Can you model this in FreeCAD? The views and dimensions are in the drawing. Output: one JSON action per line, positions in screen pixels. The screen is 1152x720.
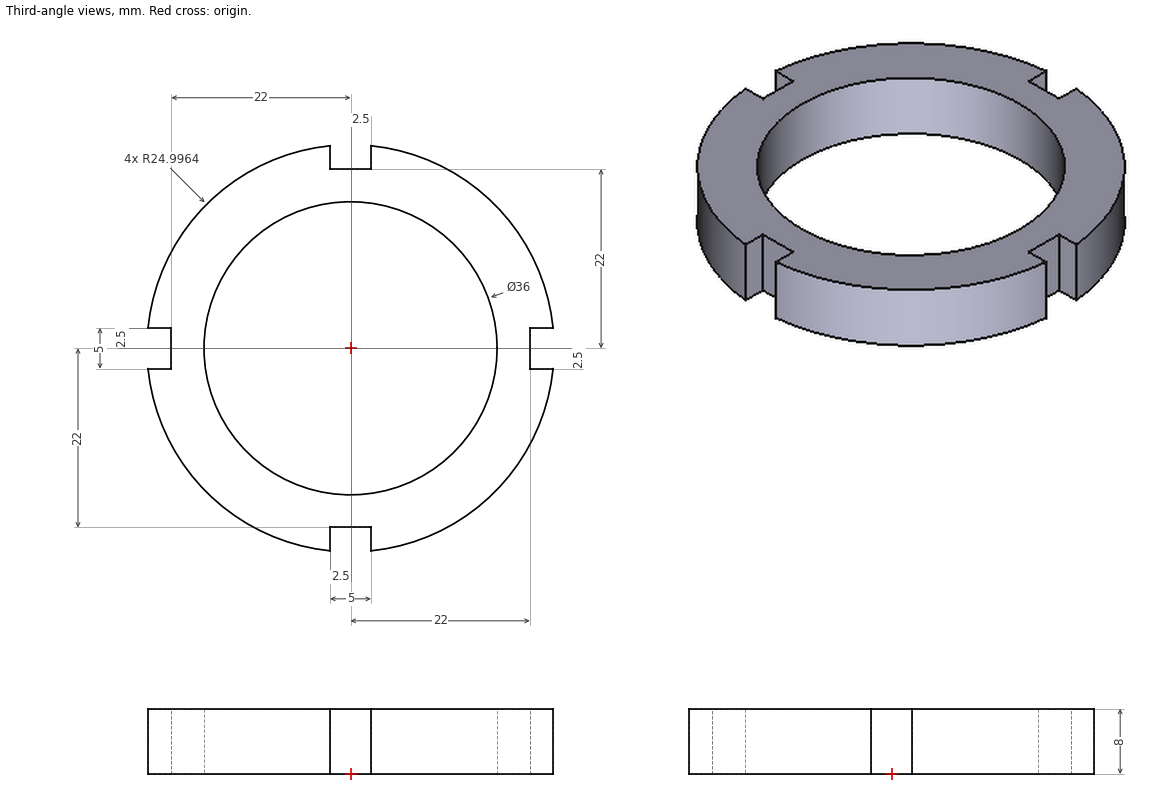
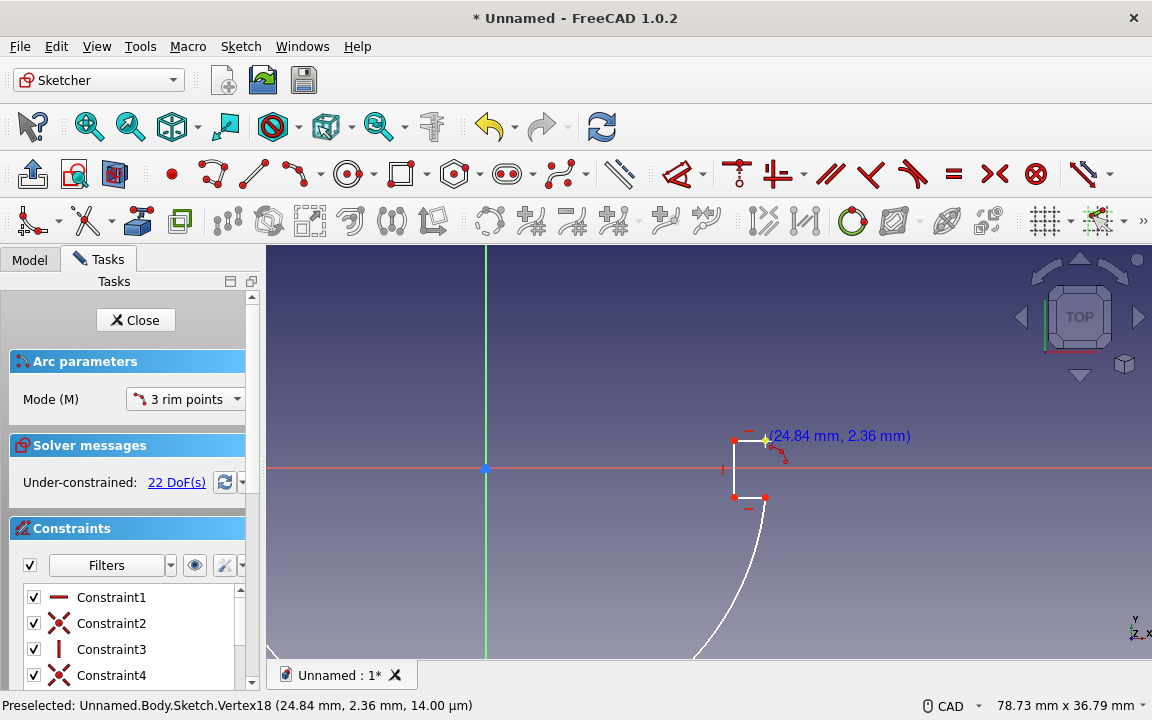
{"action": "scroll", "coordinate": [767, 439], "scroll_direction": "down", "scroll_amount": 4}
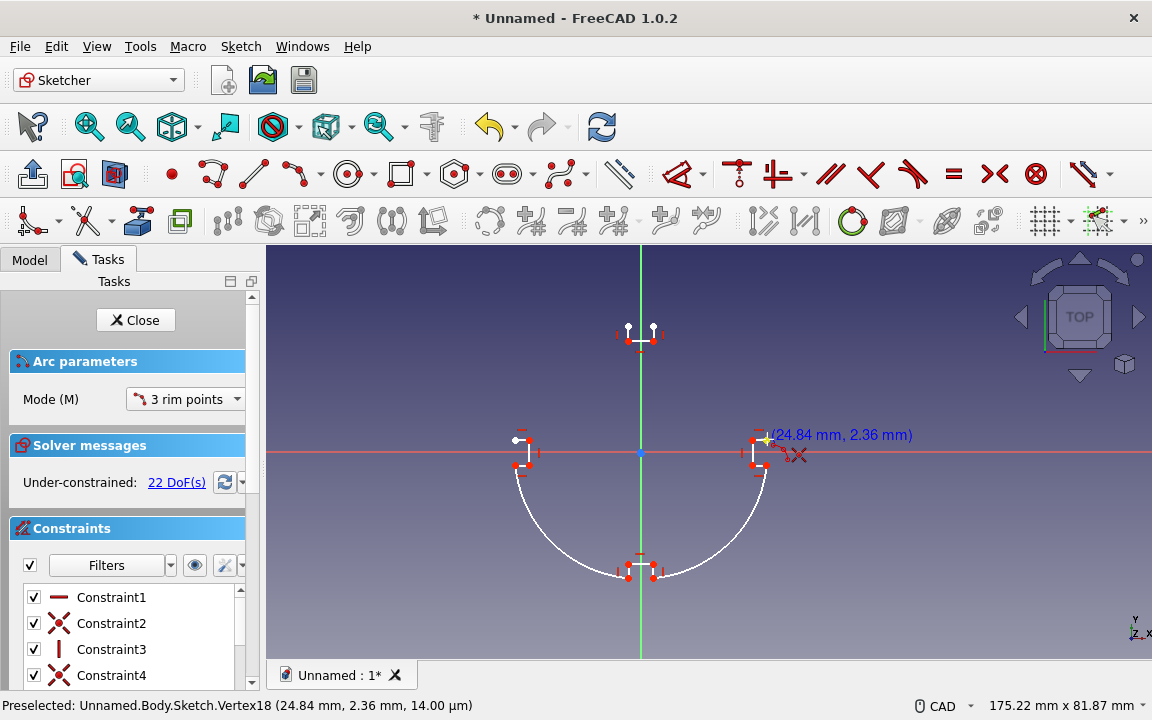
{"action": "scroll", "coordinate": [654, 326], "scroll_direction": "up", "scroll_amount": 4}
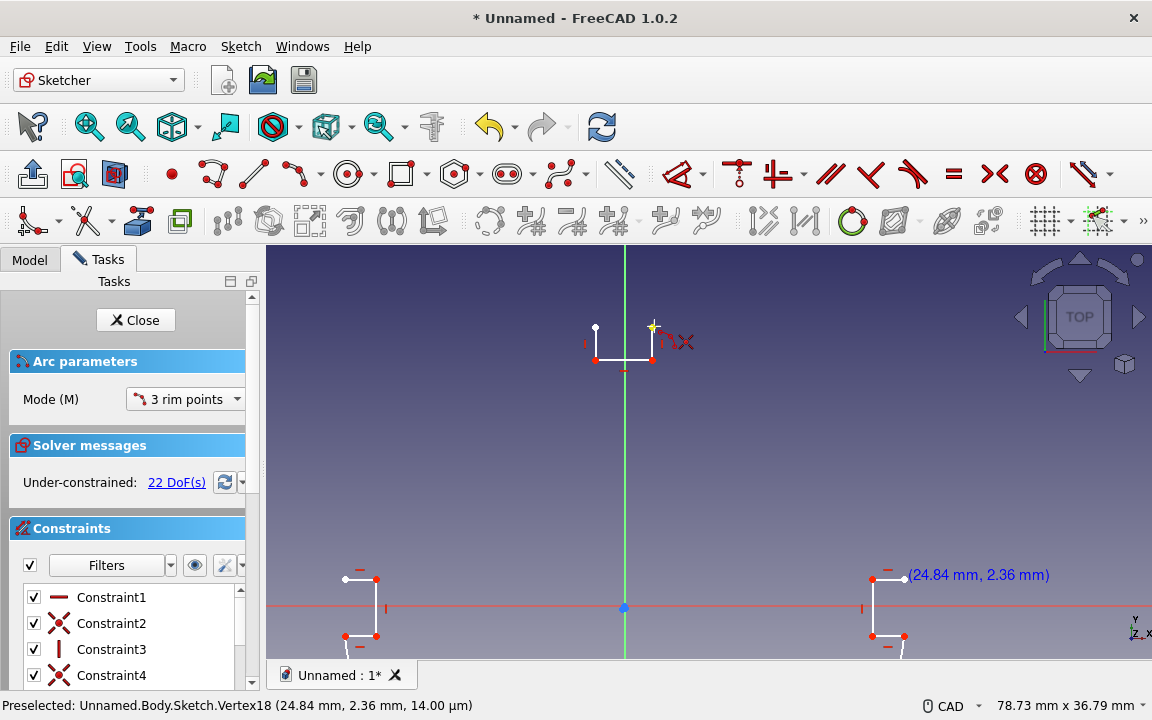
{"action": "left_click", "coordinate": [652, 327]}
{"action": "left_click", "coordinate": [823, 407]}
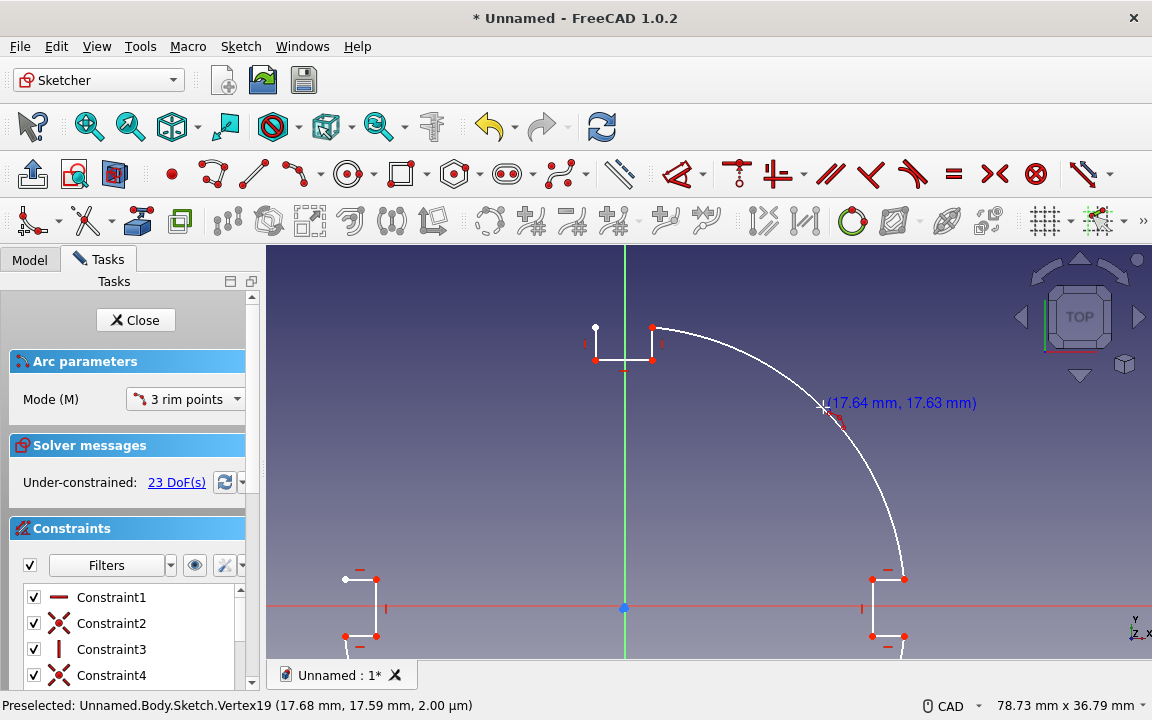
{"action": "left_click", "coordinate": [596, 327]}
{"action": "left_click", "coordinate": [345, 580]}
{"action": "left_click", "coordinate": [426, 407]}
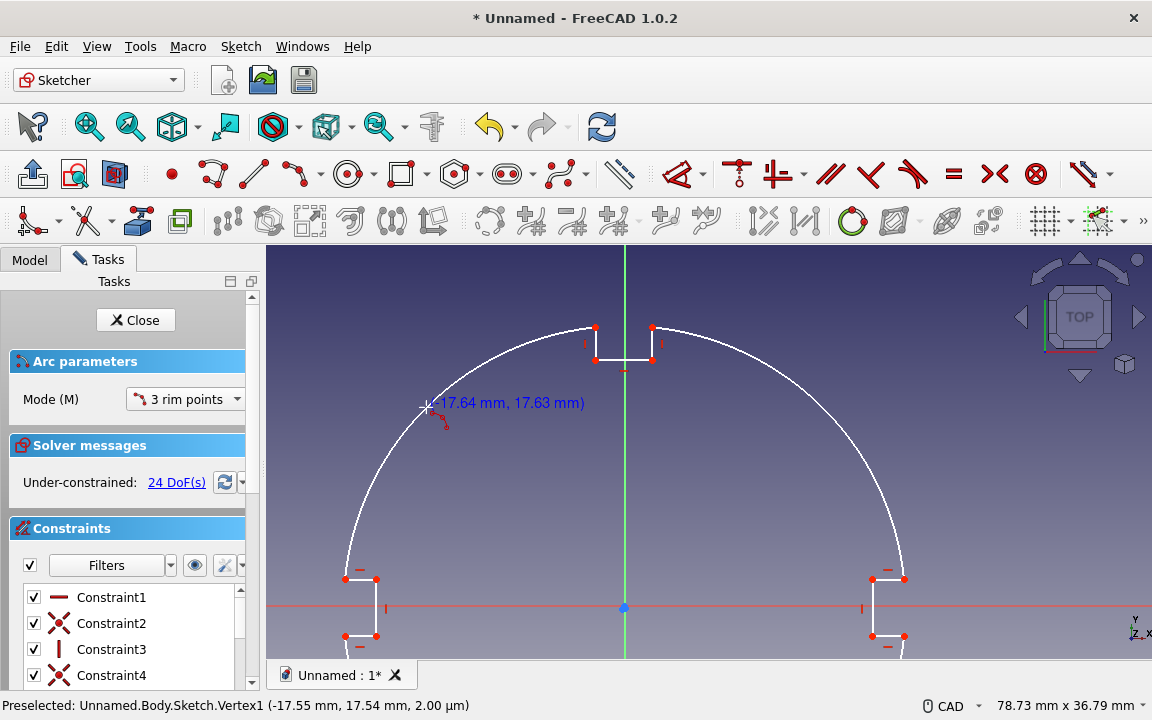
{"action": "key", "text": "g c"}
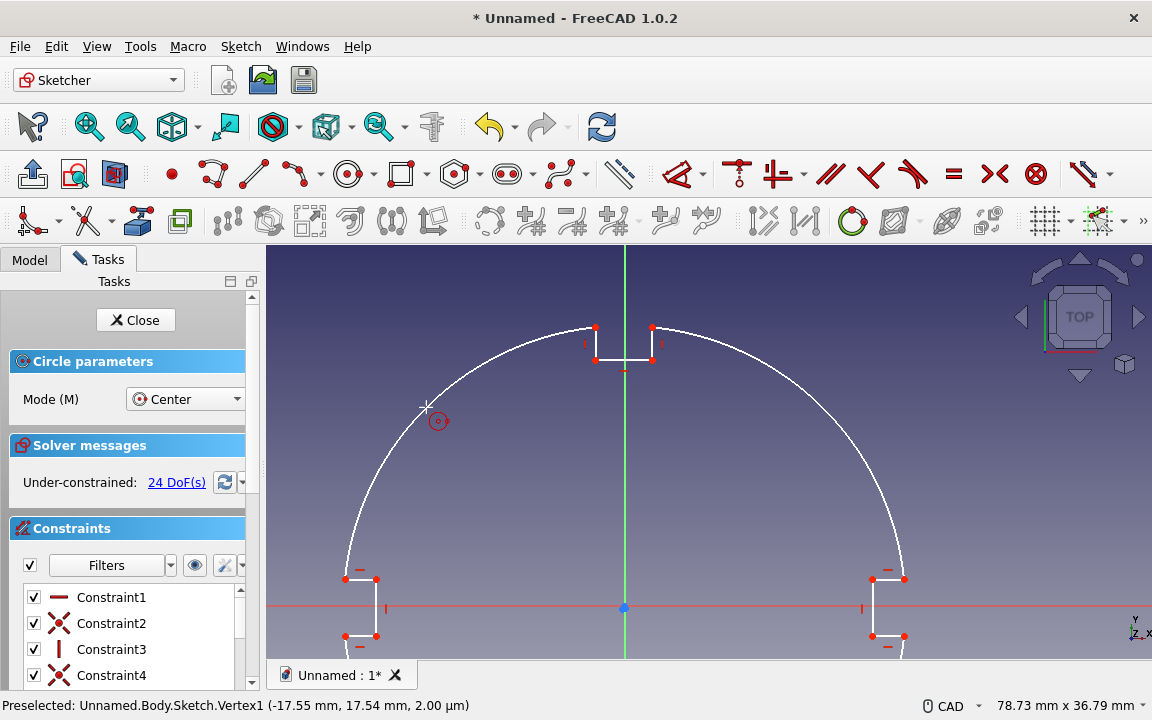
{"action": "left_click", "coordinate": [625, 606]}
{"action": "mouse_move", "coordinate": [768, 463]}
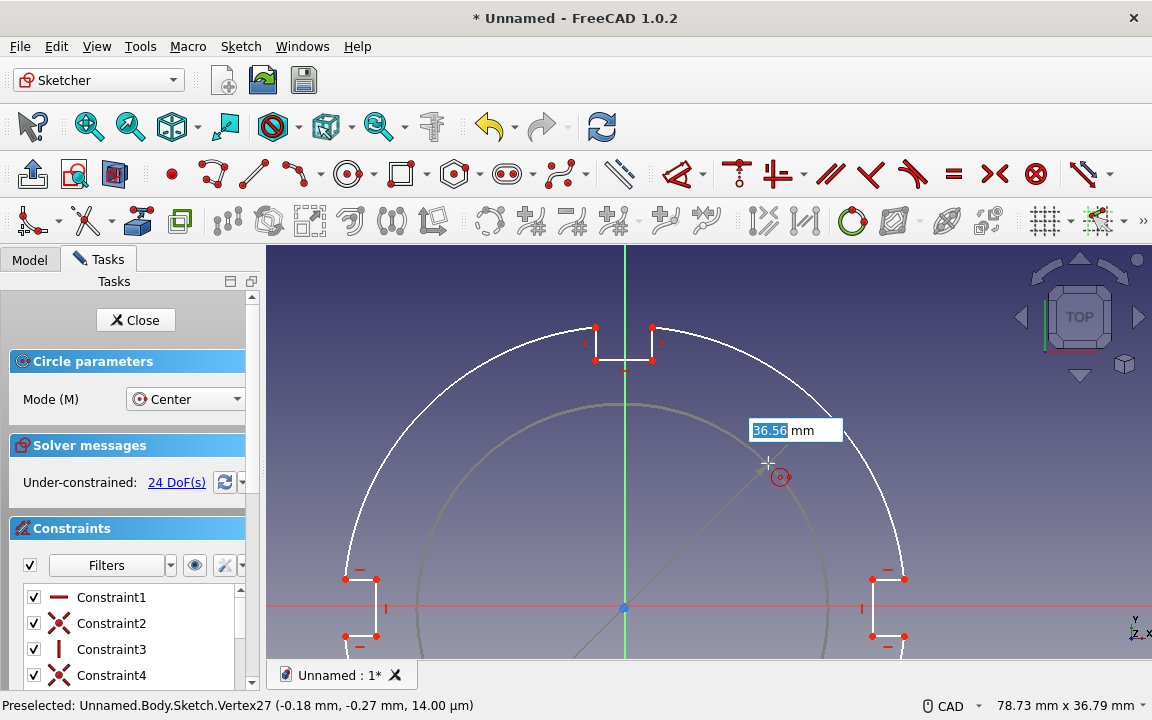
{"action": "type", "text": "36"}
{"action": "key", "text": "Return"}
{"action": "key", "text": "Escape"}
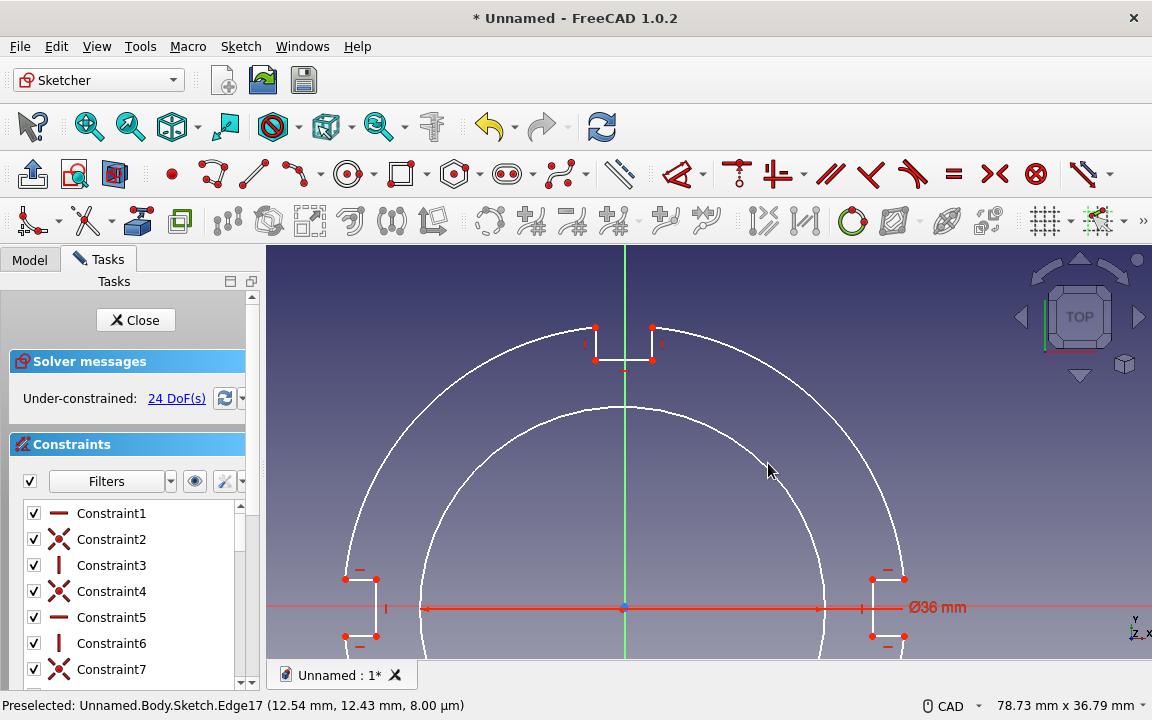
{"action": "left_click", "coordinate": [765, 466]}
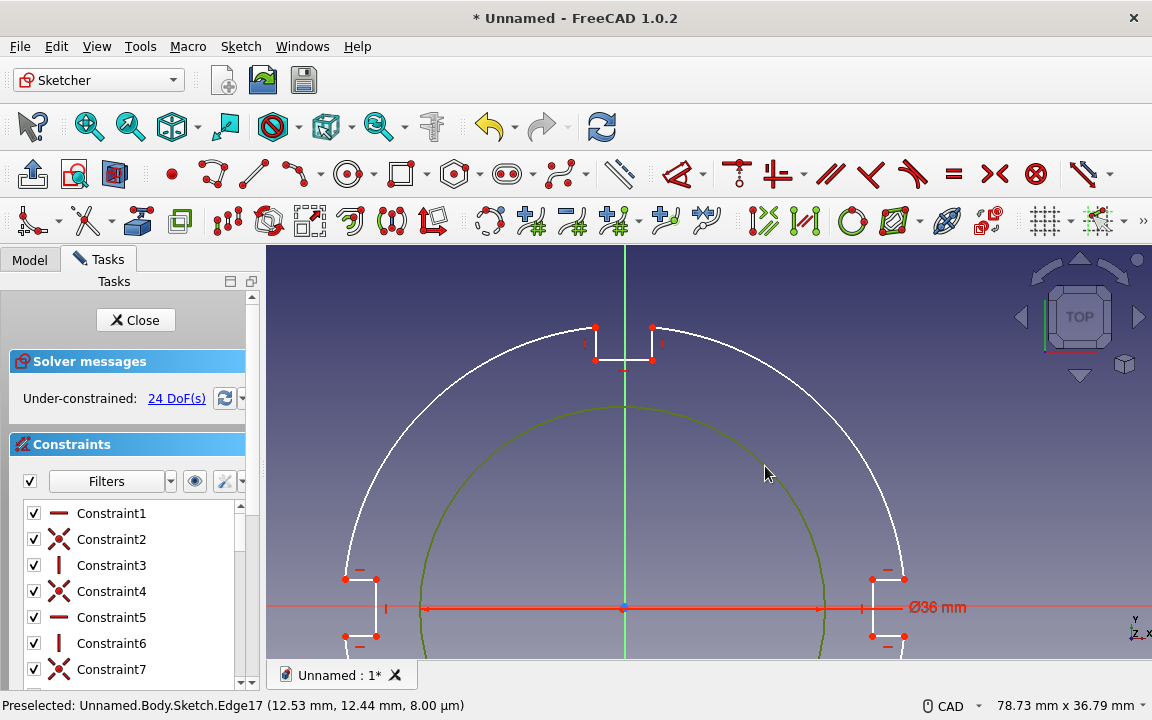
{"action": "scroll", "coordinate": [654, 326], "scroll_direction": "down", "scroll_amount": 4}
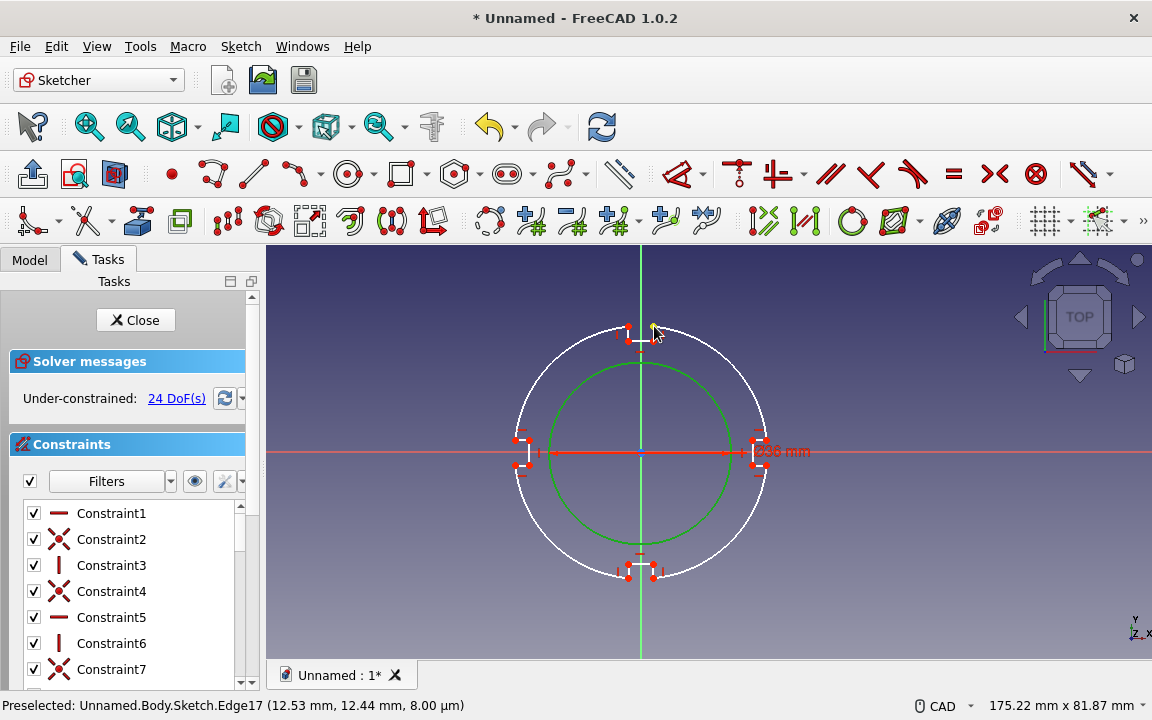
{"action": "left_click", "coordinate": [703, 563]}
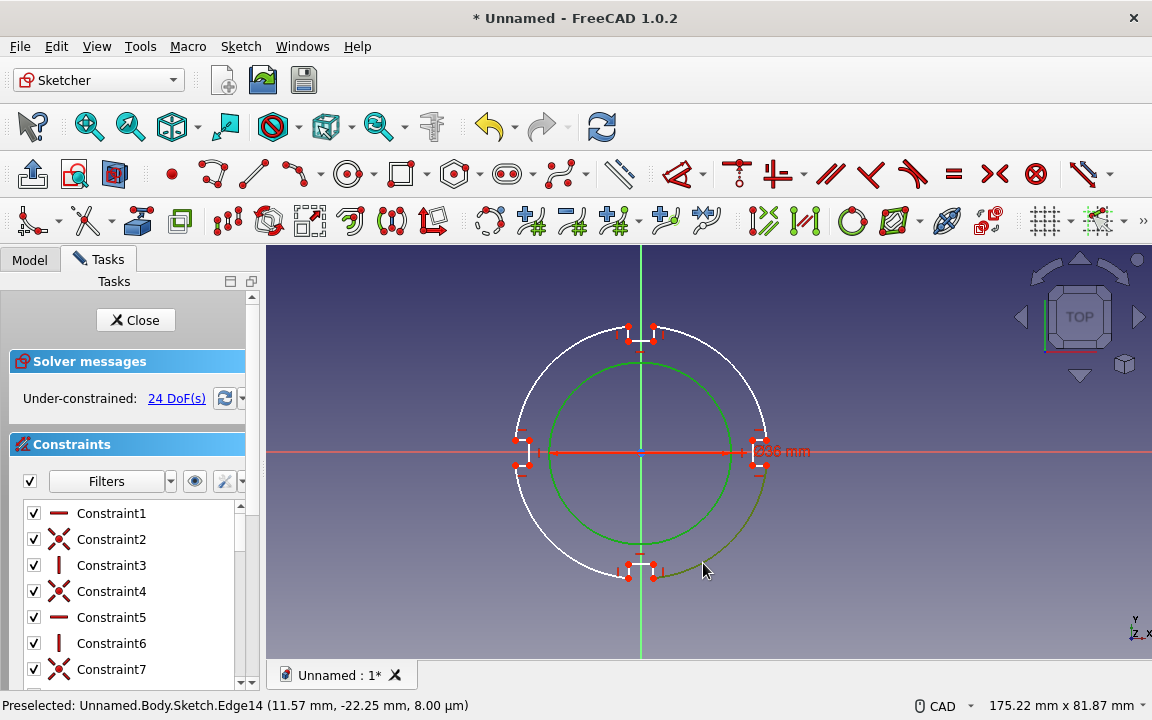
{"action": "key", "text": "c"}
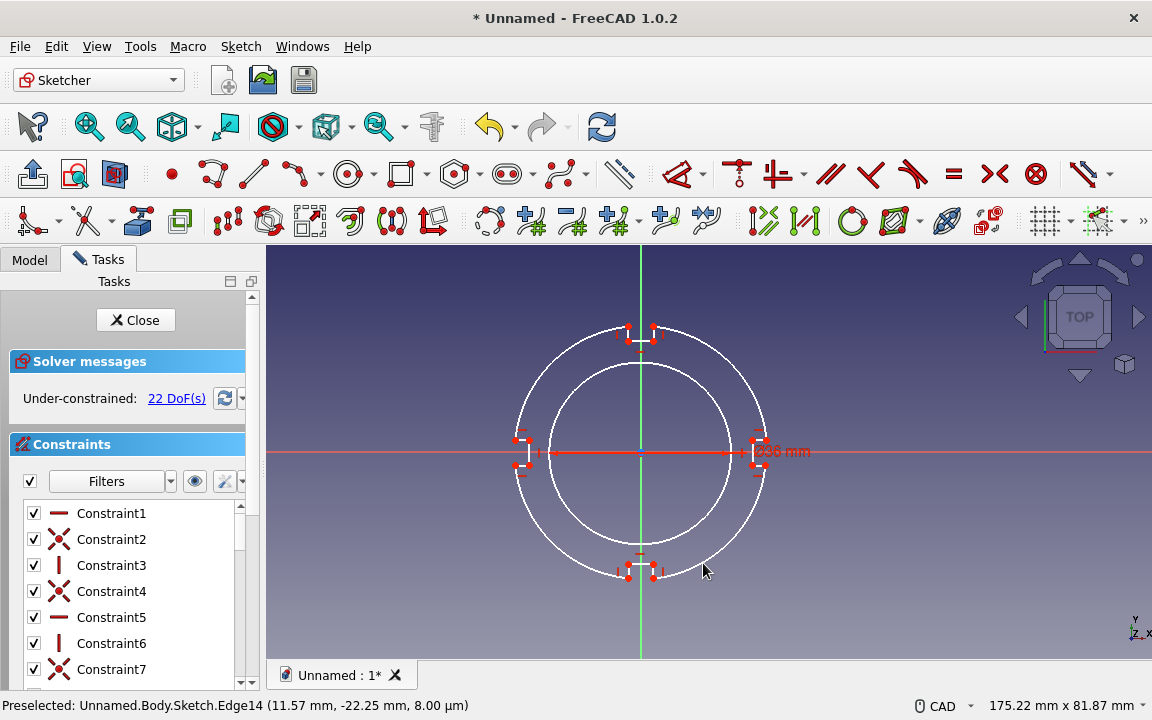
{"action": "left_click", "coordinate": [704, 389]}